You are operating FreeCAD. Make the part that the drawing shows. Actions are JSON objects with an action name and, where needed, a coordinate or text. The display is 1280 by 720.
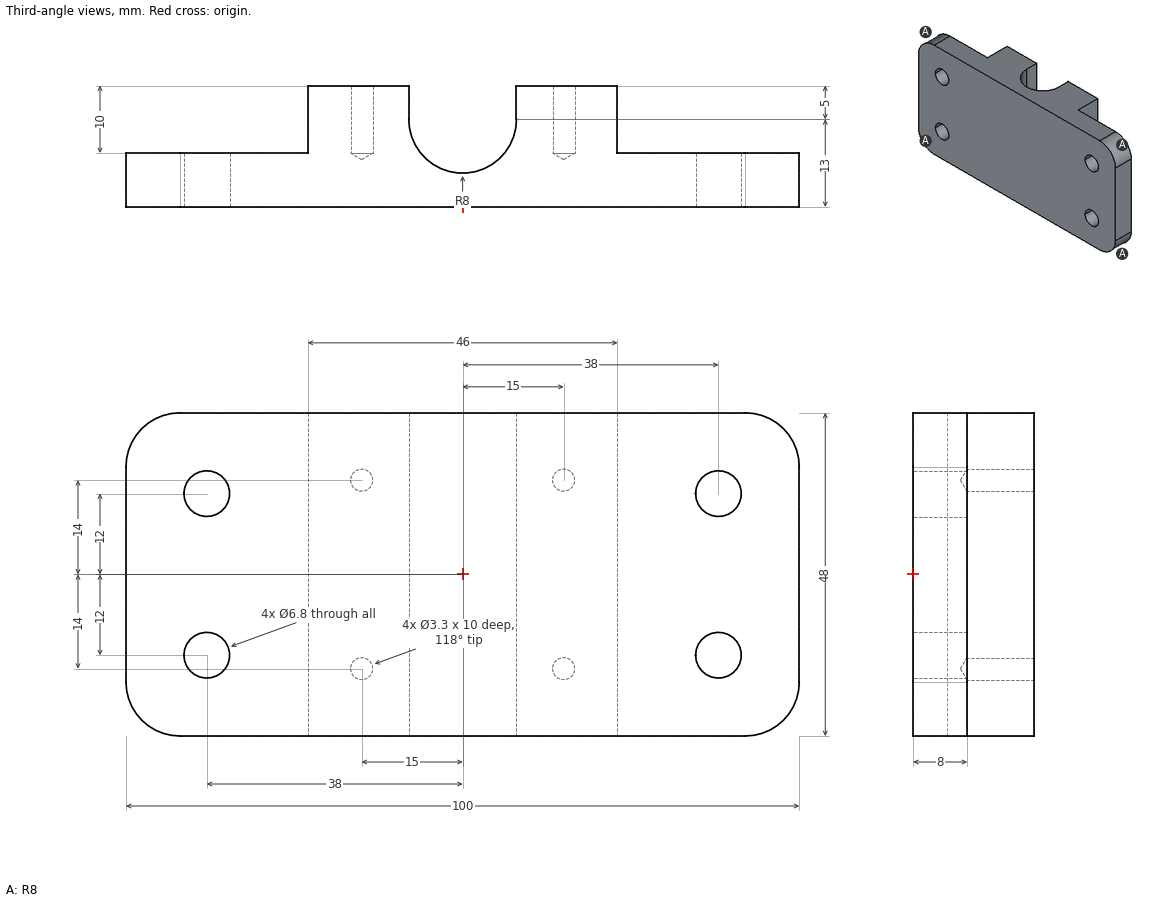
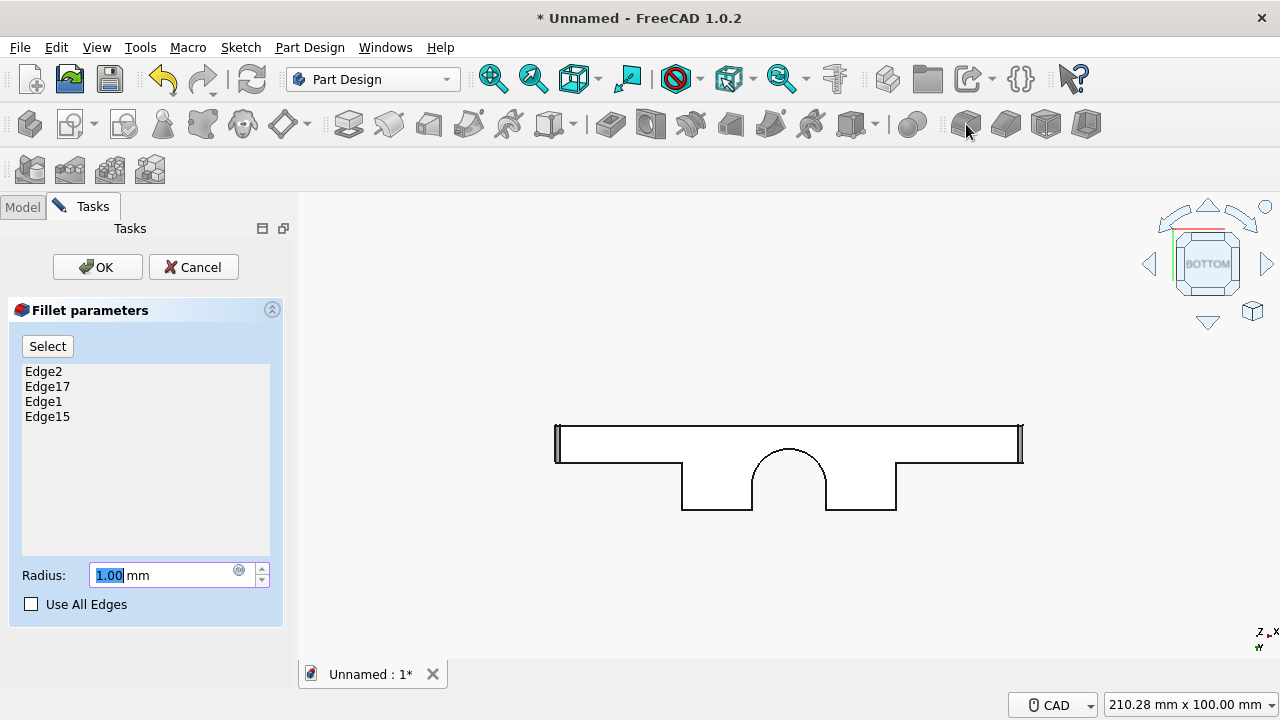
{"action": "type", "text": "8"}
{"action": "key", "text": "Tab"}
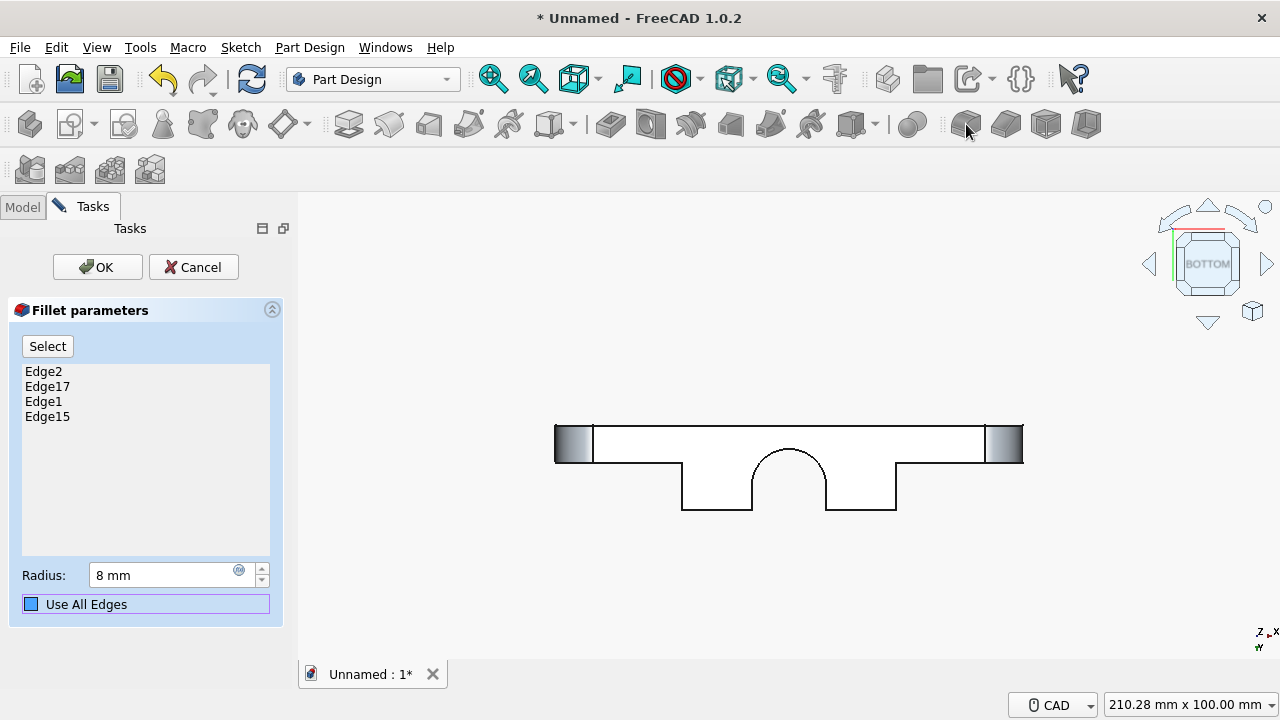
{"action": "left_click", "coordinate": [98, 267]}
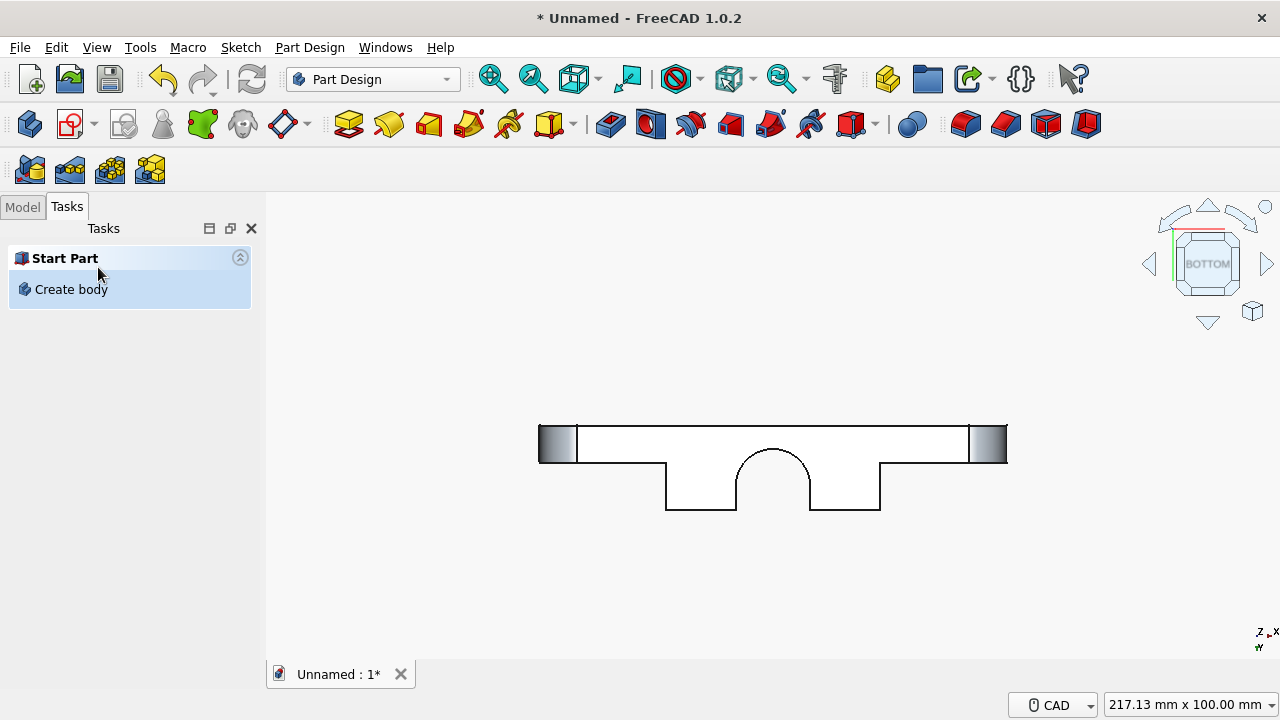
{"action": "key", "text": "4"}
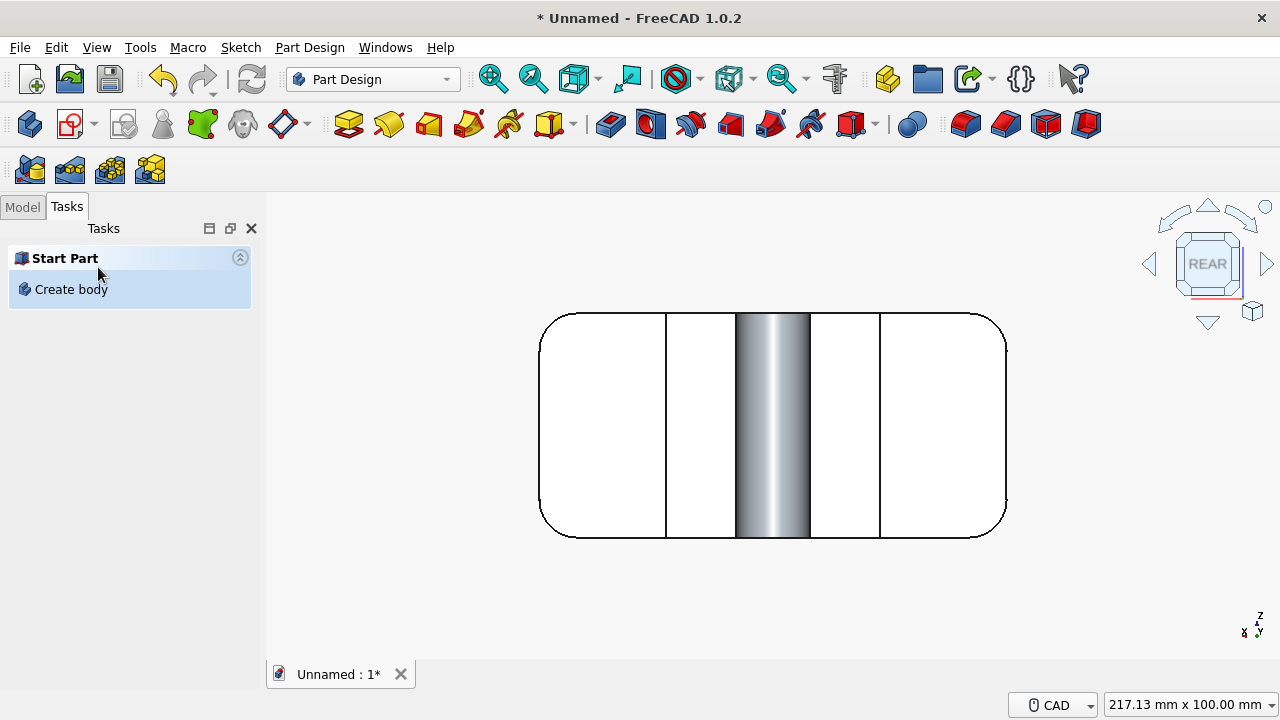
{"action": "left_click", "coordinate": [845, 360]}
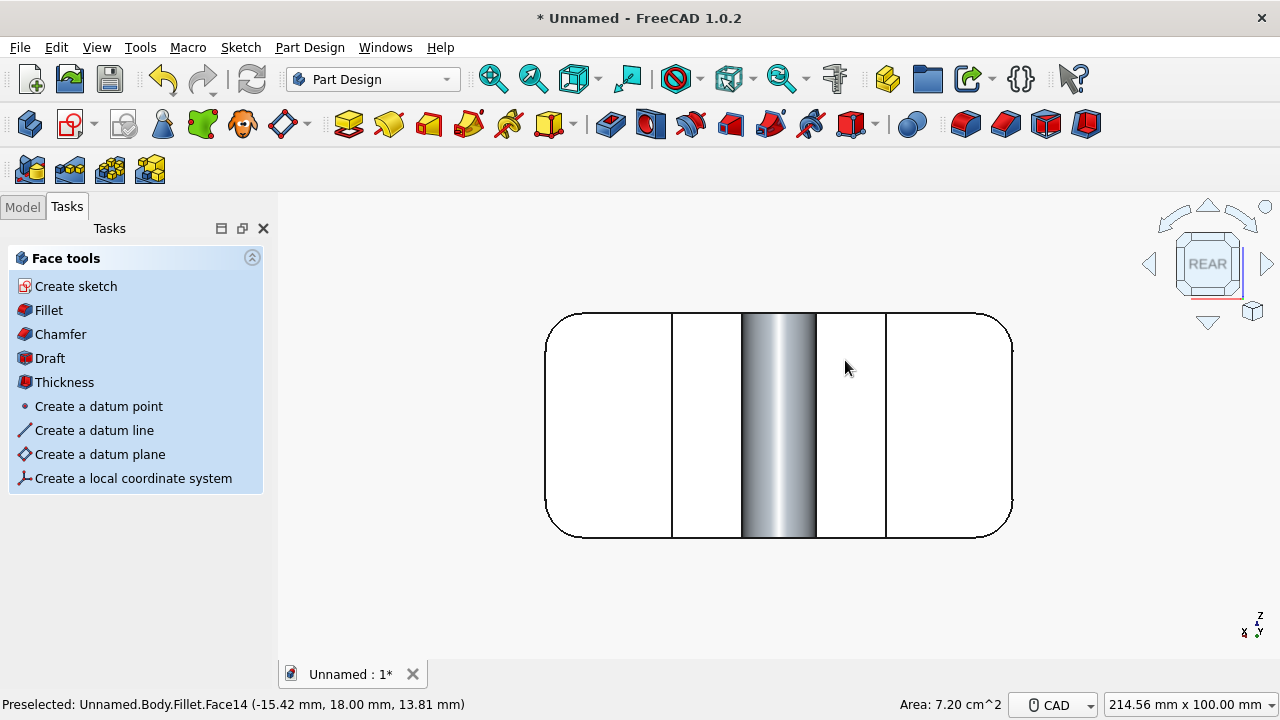
{"action": "left_click", "coordinate": [70, 124]}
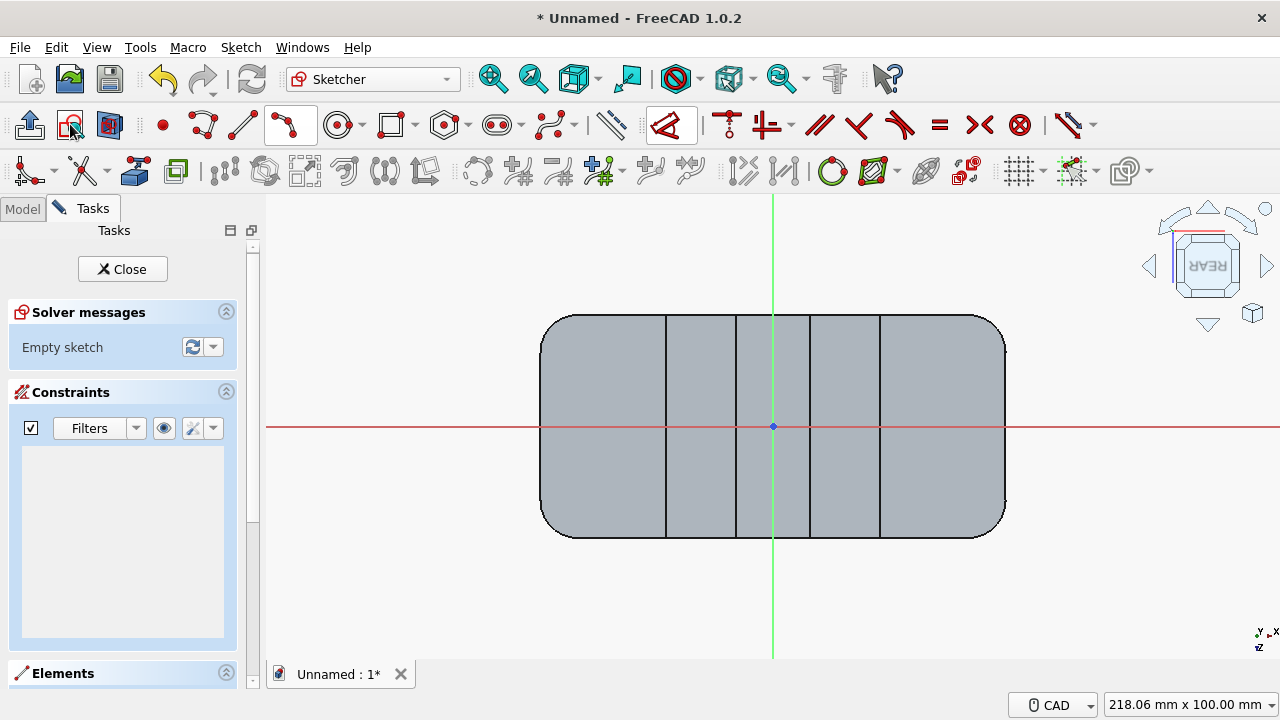
{"action": "scroll", "coordinate": [856, 427], "scroll_direction": "up", "scroll_amount": 3}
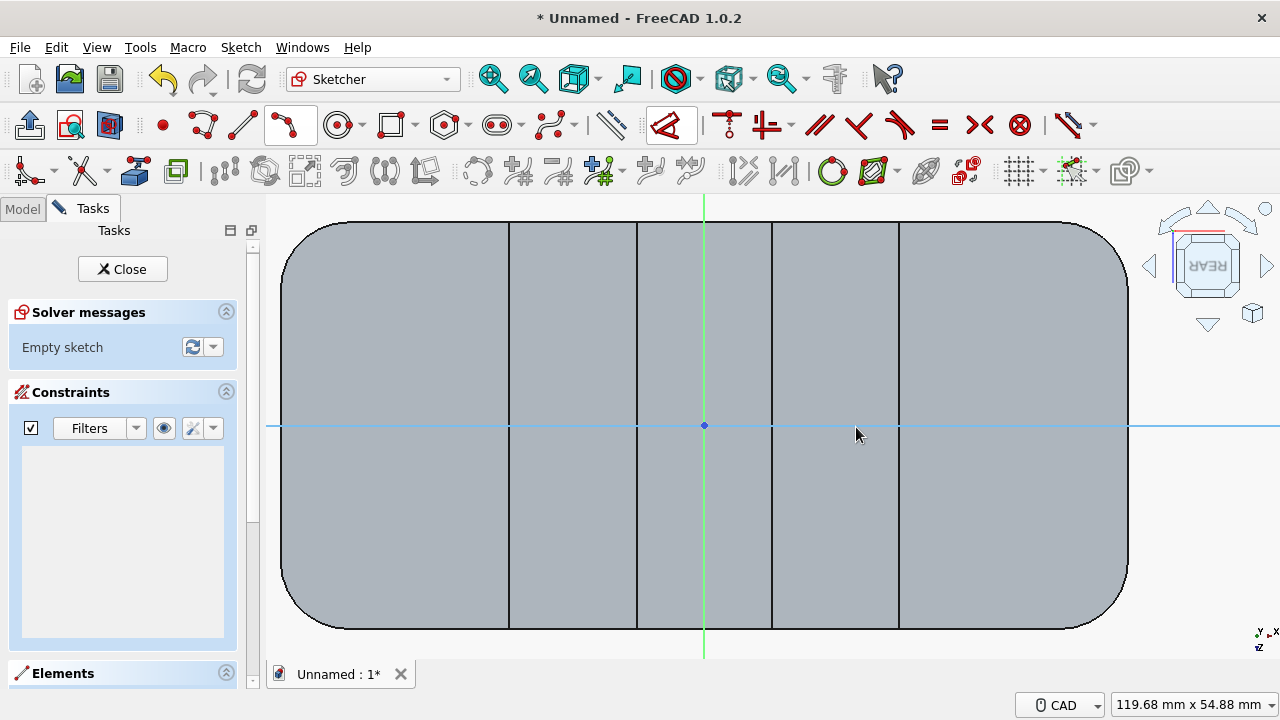
{"action": "left_click", "coordinate": [338, 126]}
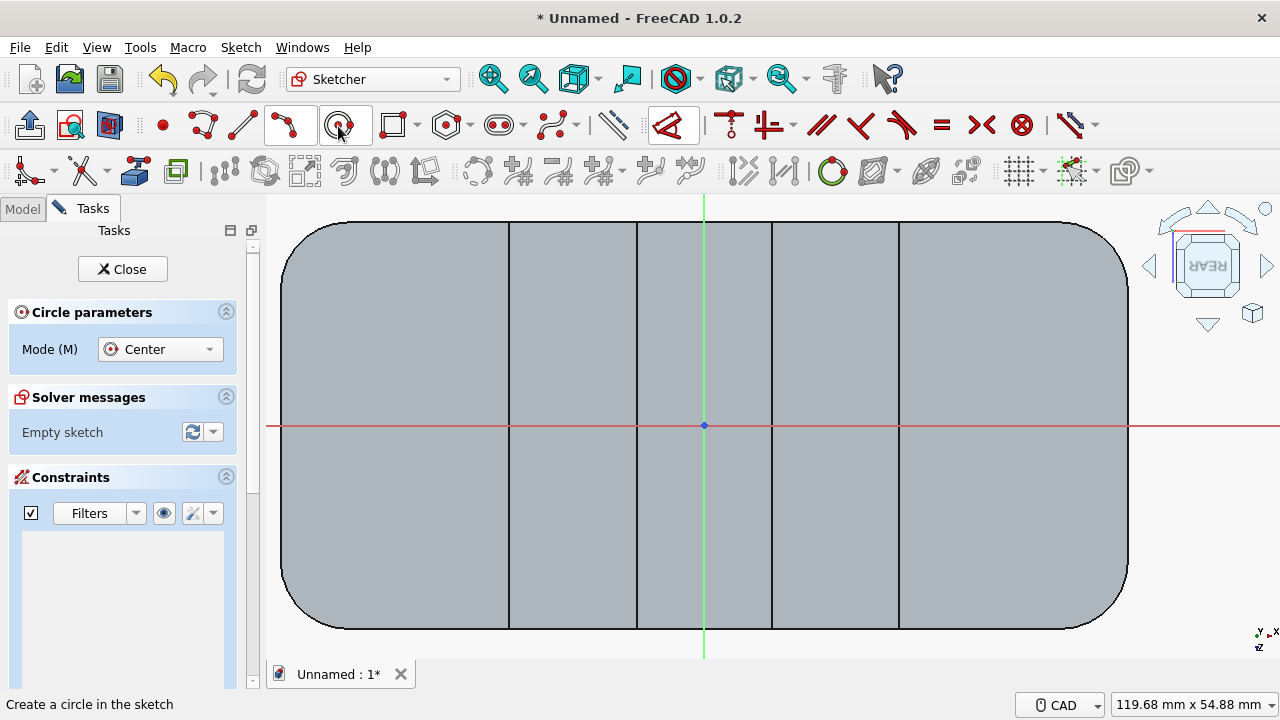
{"action": "scroll", "coordinate": [577, 307], "scroll_direction": "up", "scroll_amount": 3}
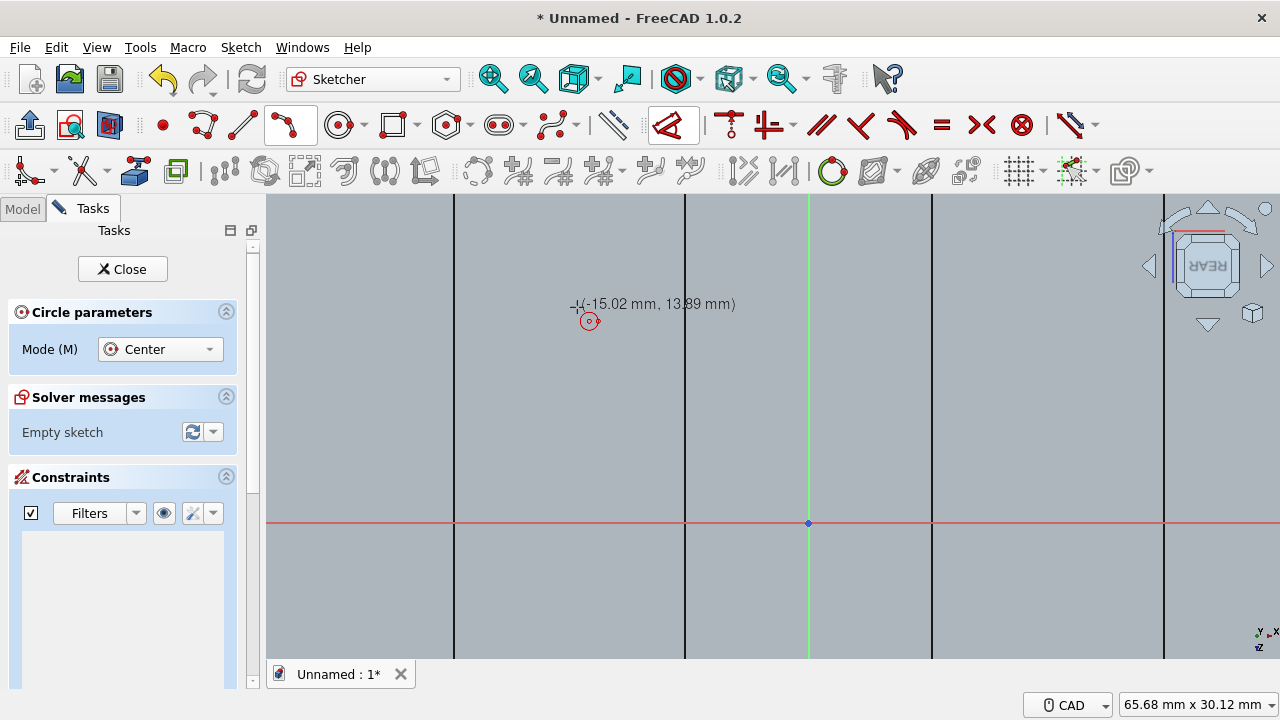
{"action": "left_click", "coordinate": [577, 307]}
{"action": "left_click", "coordinate": [595, 289]}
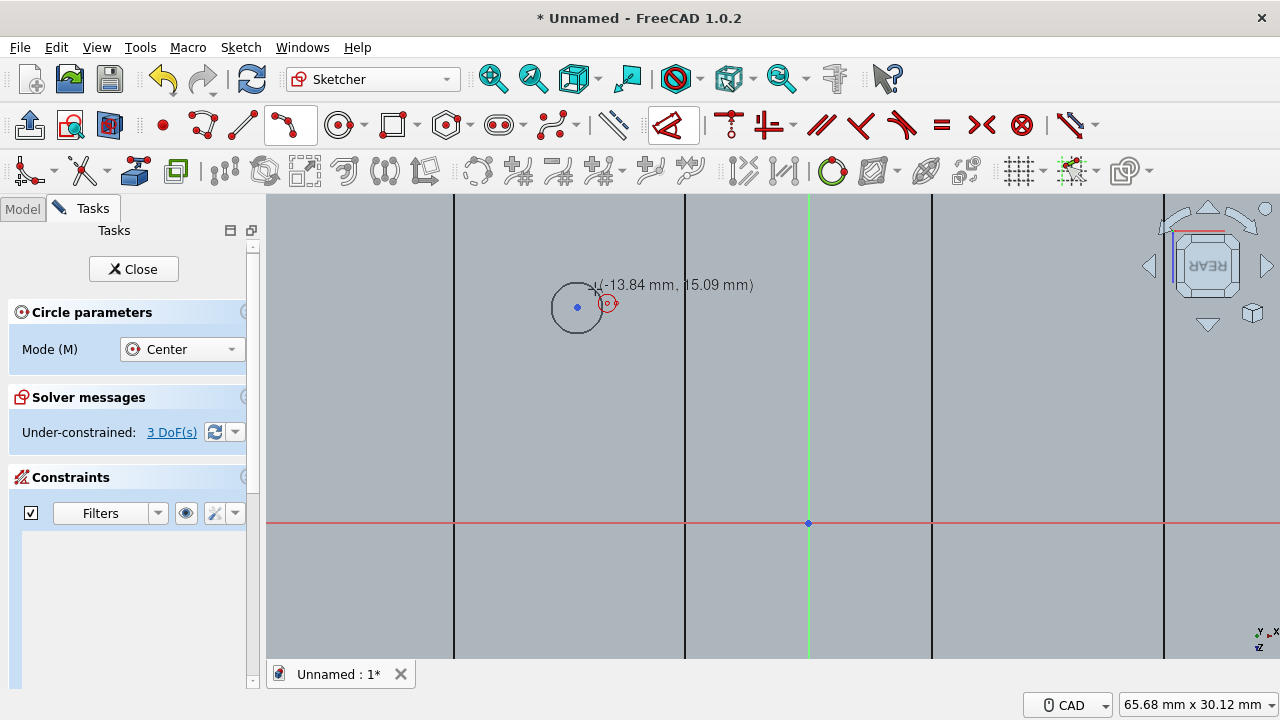
{"action": "scroll", "coordinate": [578, 309], "scroll_direction": "down", "scroll_amount": 3}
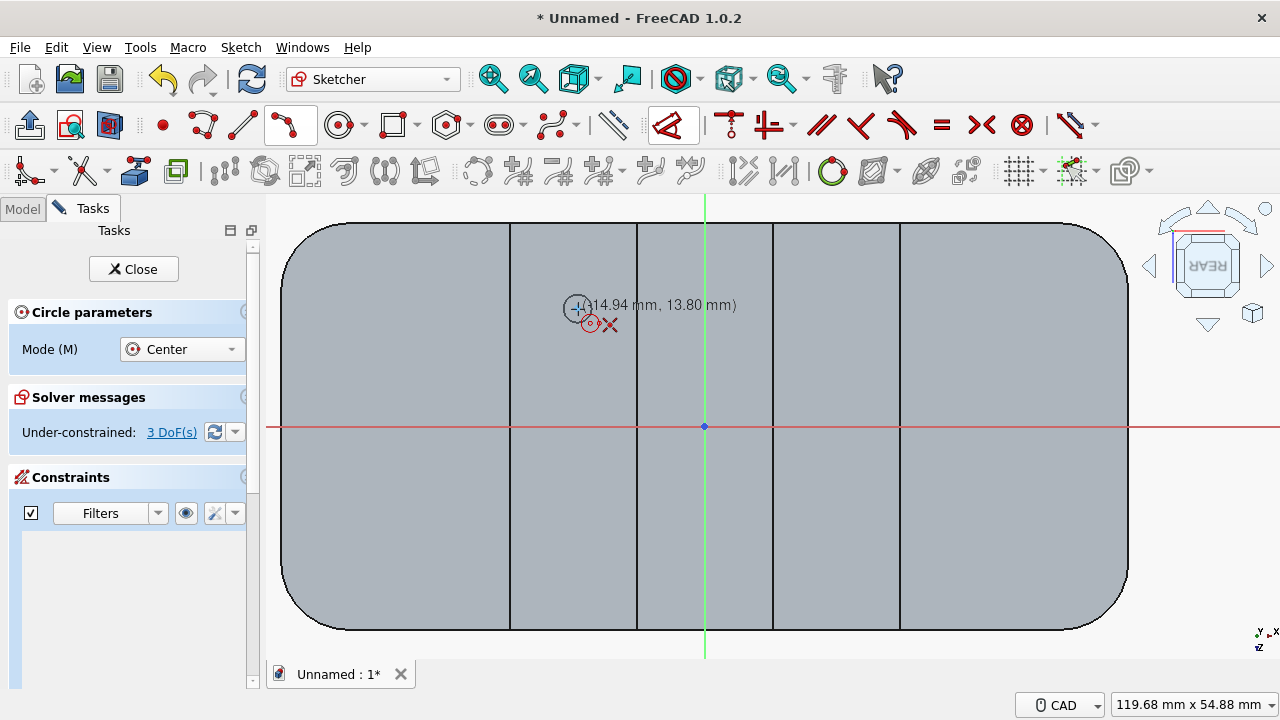
{"action": "scroll", "coordinate": [578, 545], "scroll_direction": "up", "scroll_amount": 3}